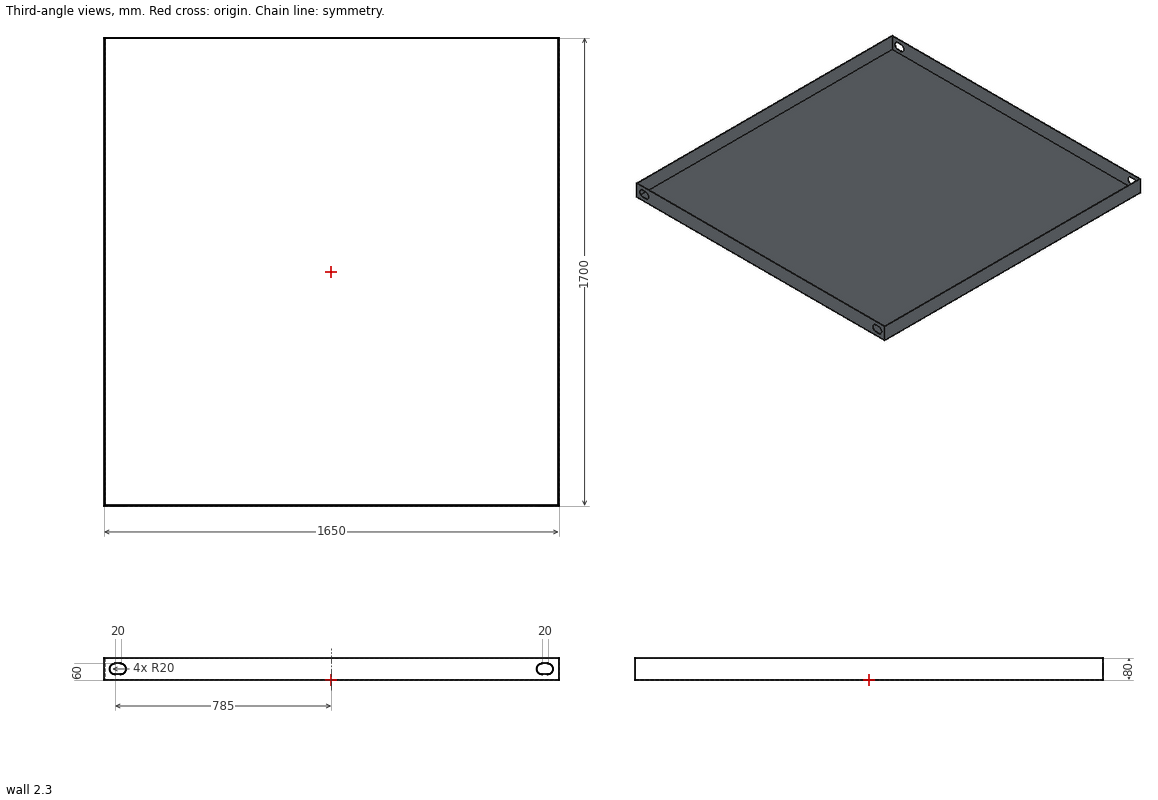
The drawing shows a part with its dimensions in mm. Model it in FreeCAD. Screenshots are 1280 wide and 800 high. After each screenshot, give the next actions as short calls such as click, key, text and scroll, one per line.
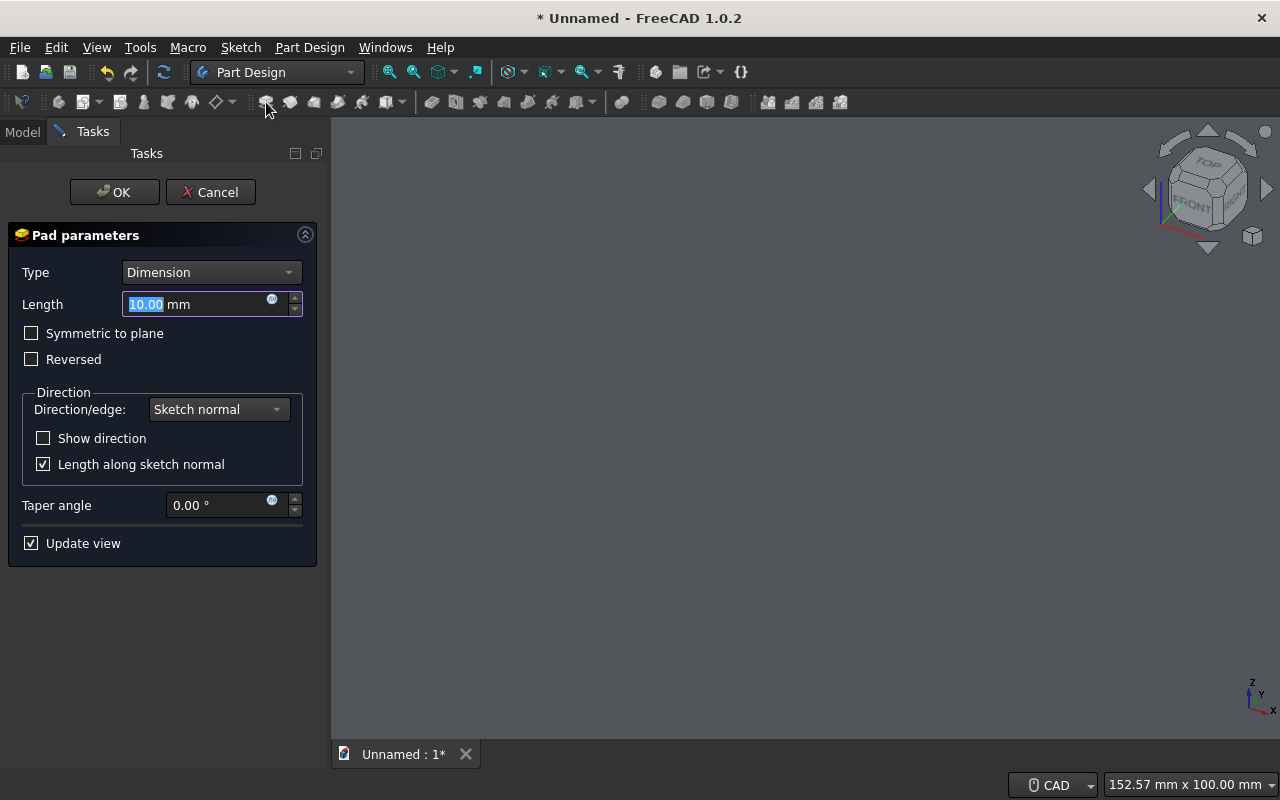
text(80)
key(Tab)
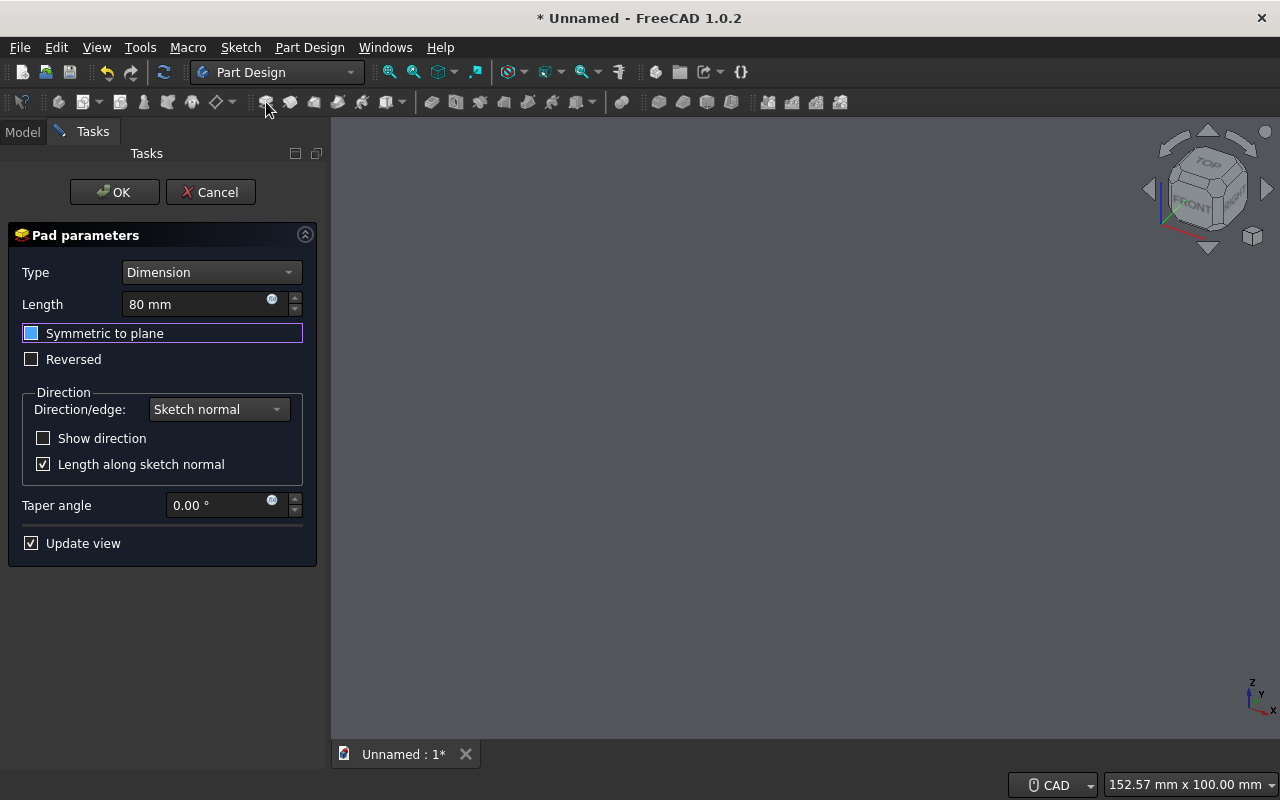
click(115, 192)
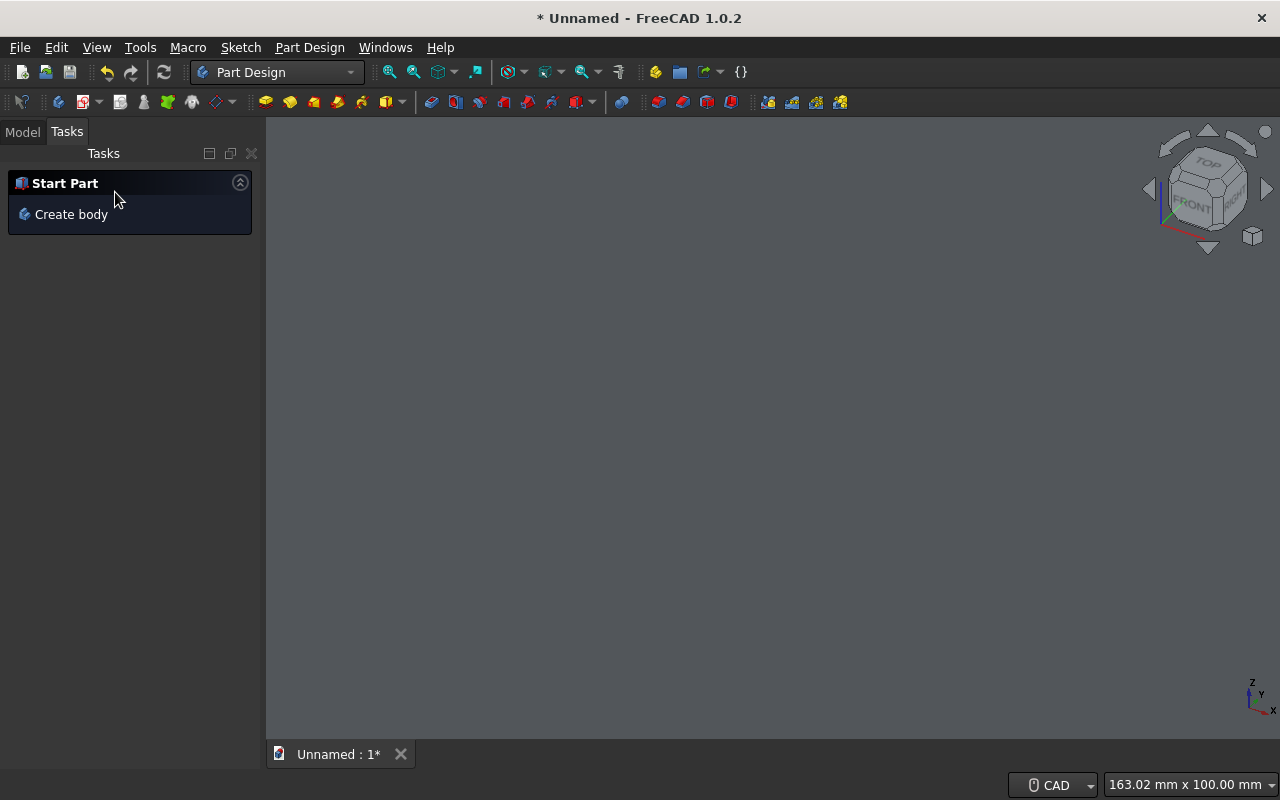
key(v)
key(f)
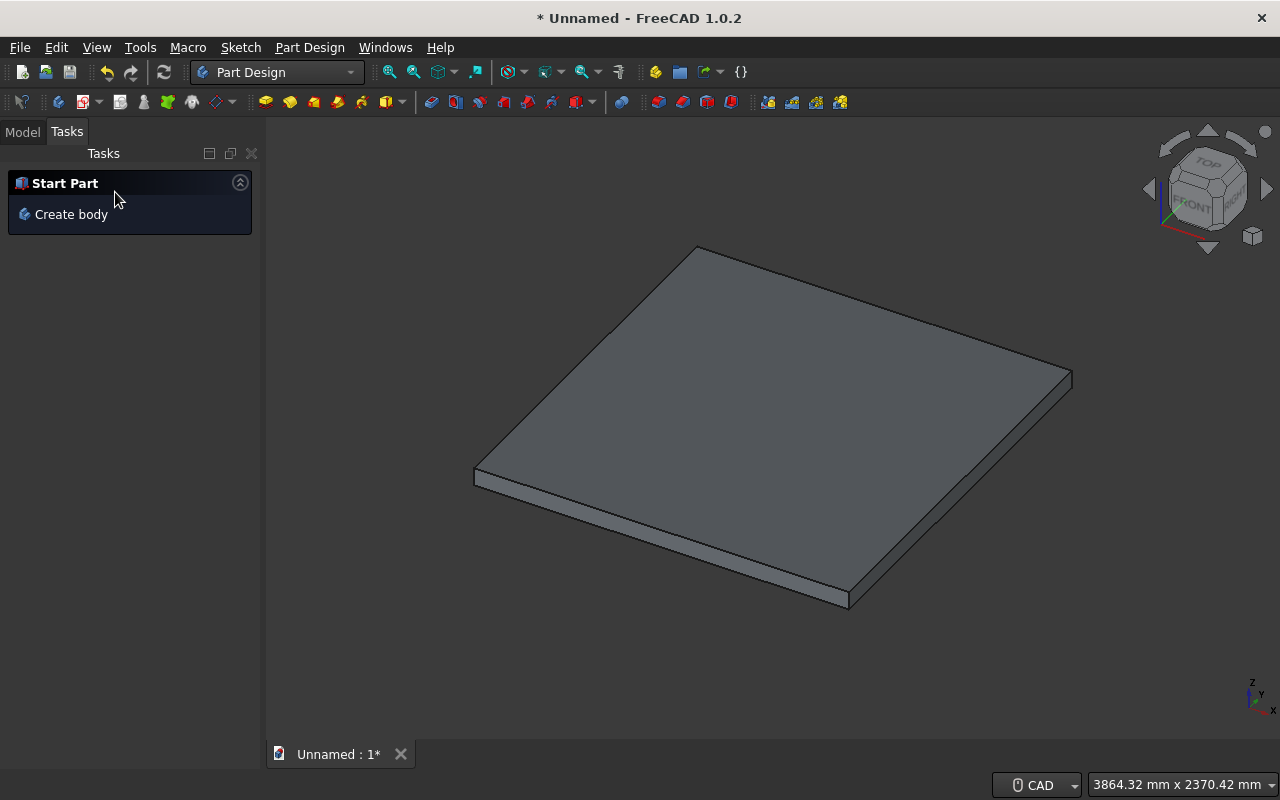
click(773, 418)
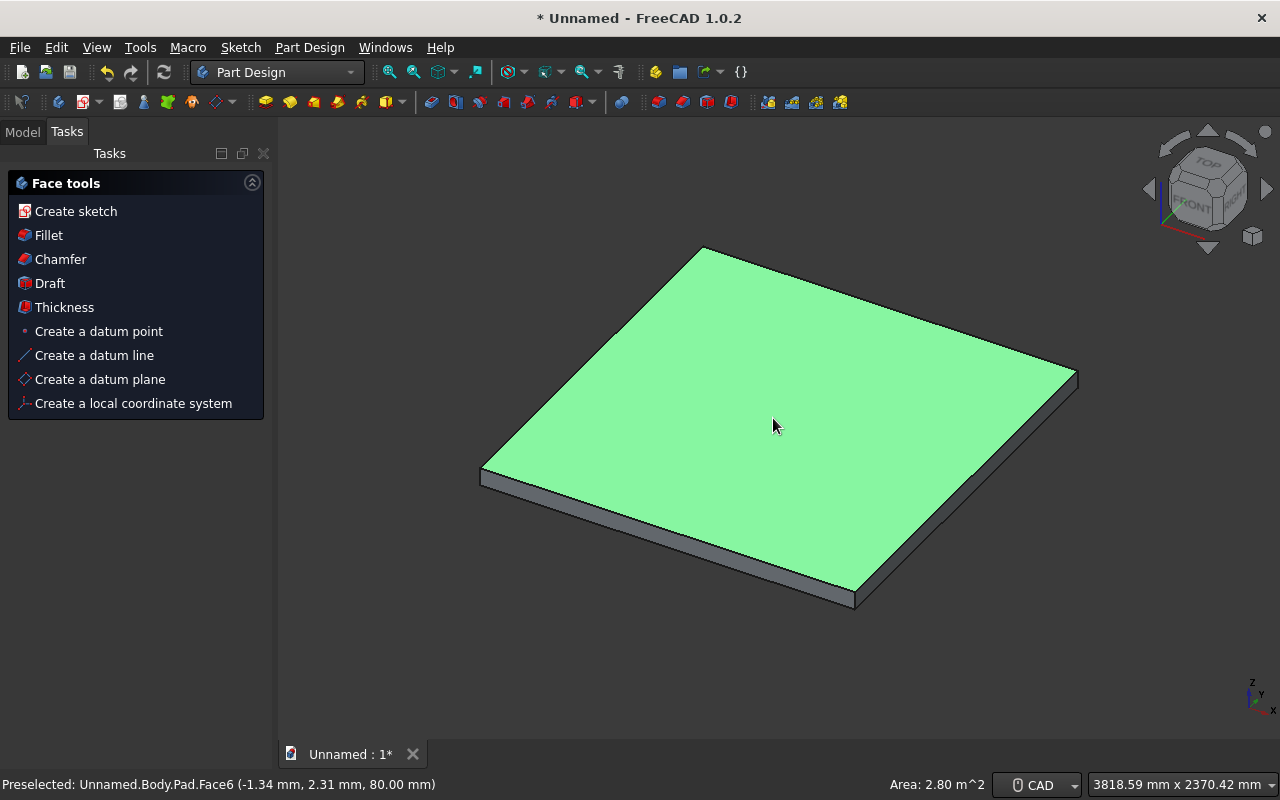
click(732, 102)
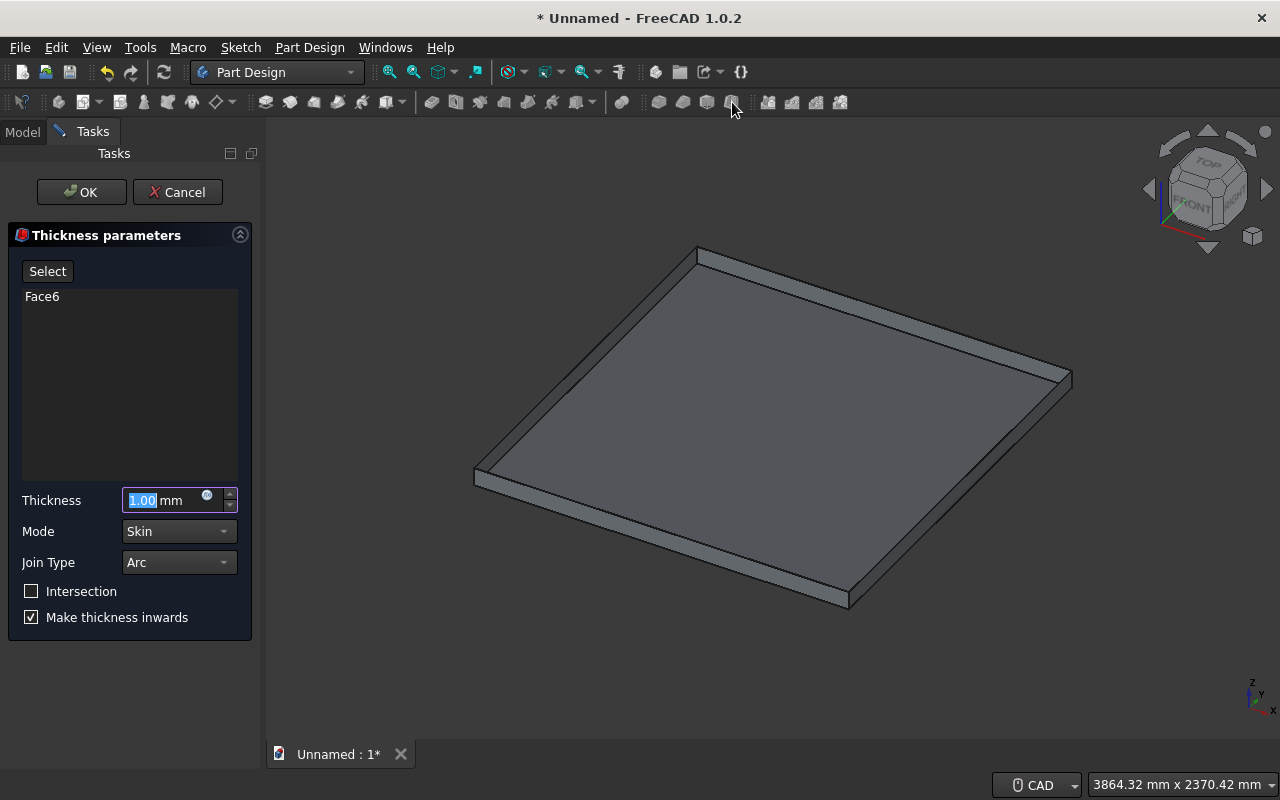
text(2.3)
key(Tab)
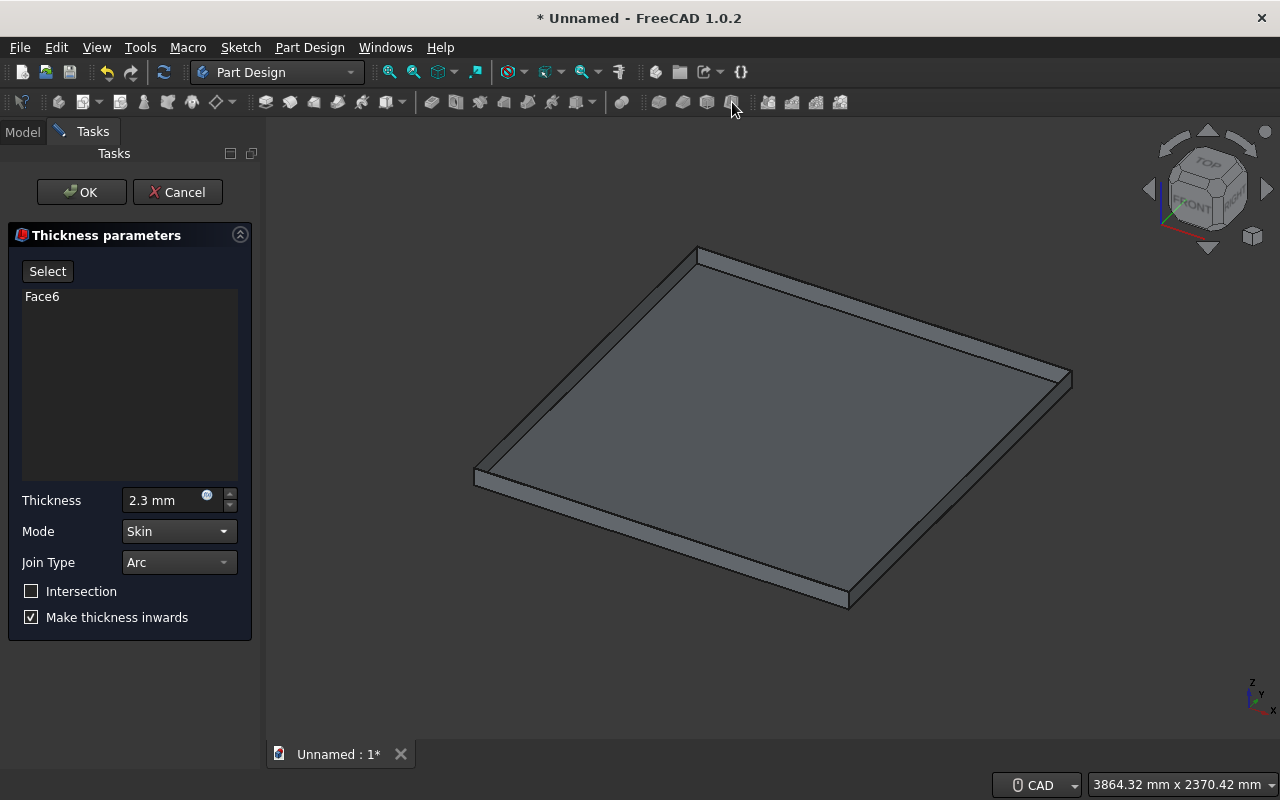
click(180, 562)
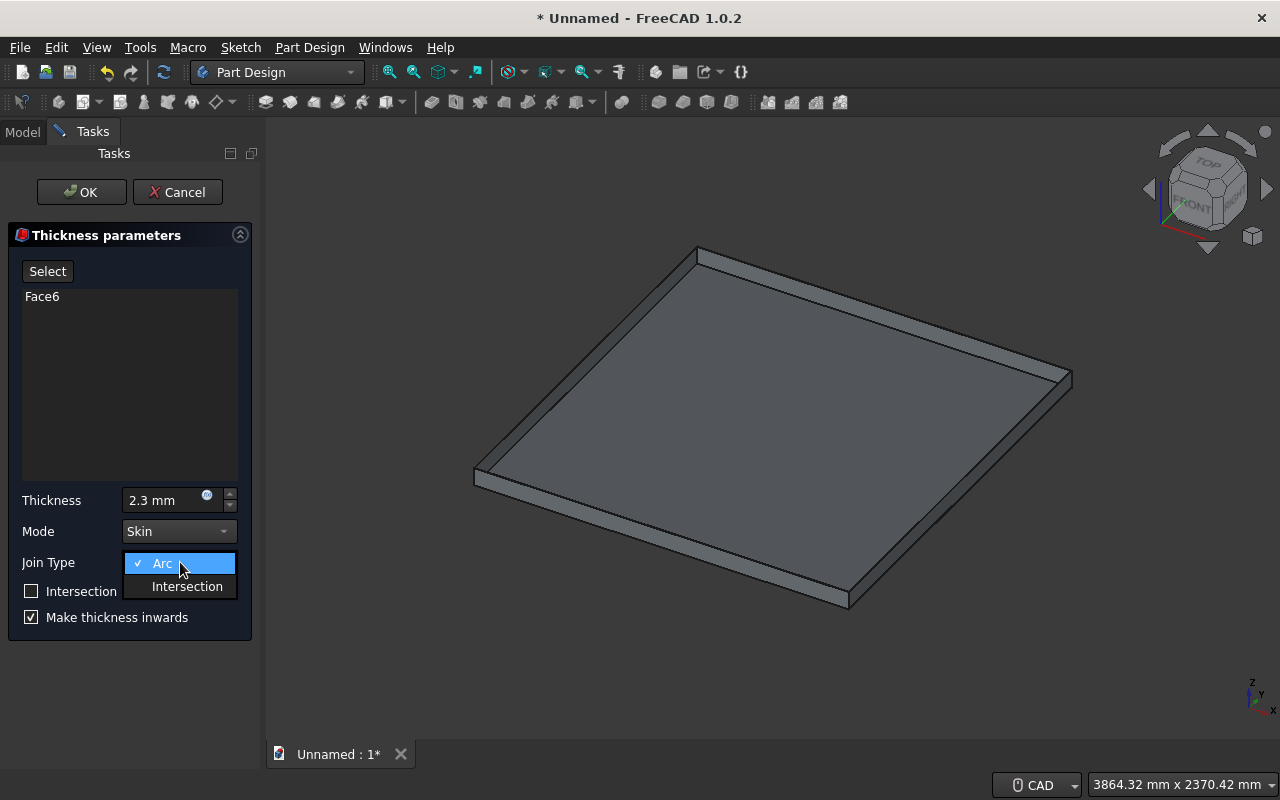
click(179, 586)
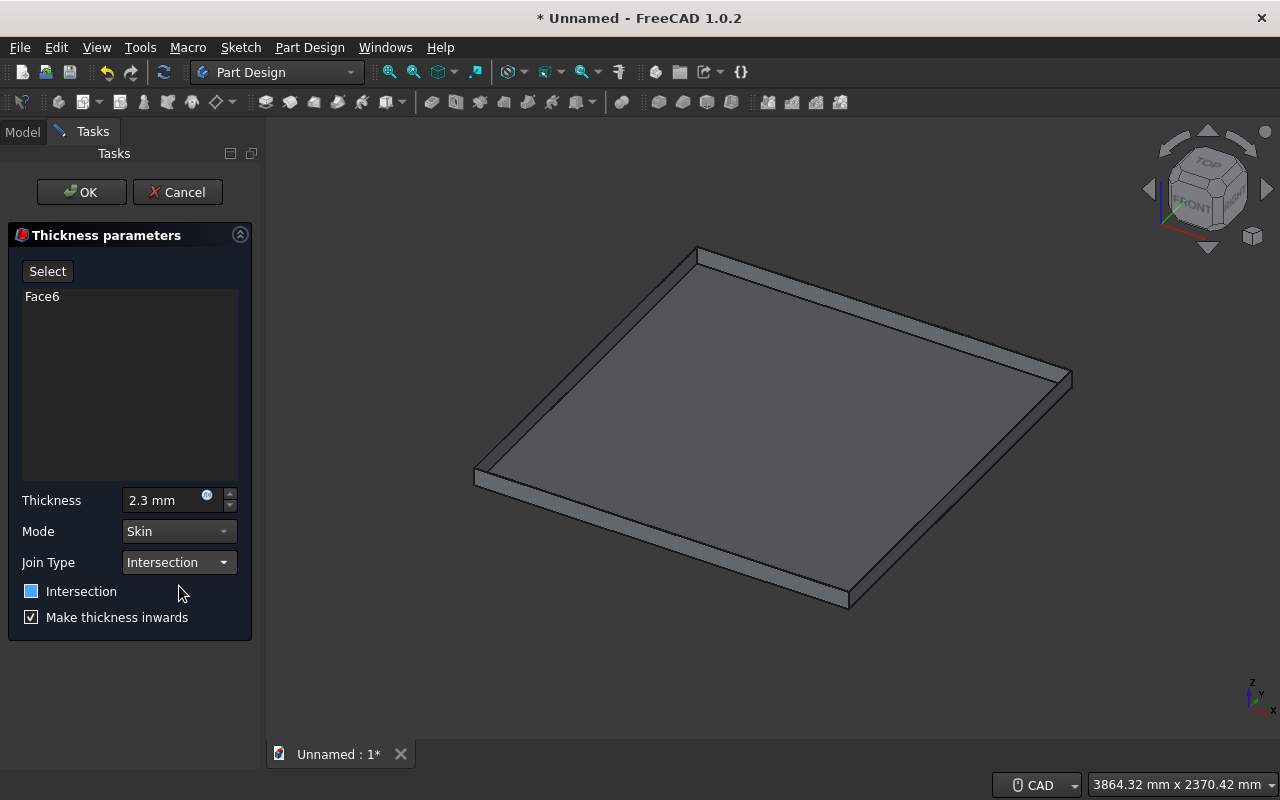
click(82, 192)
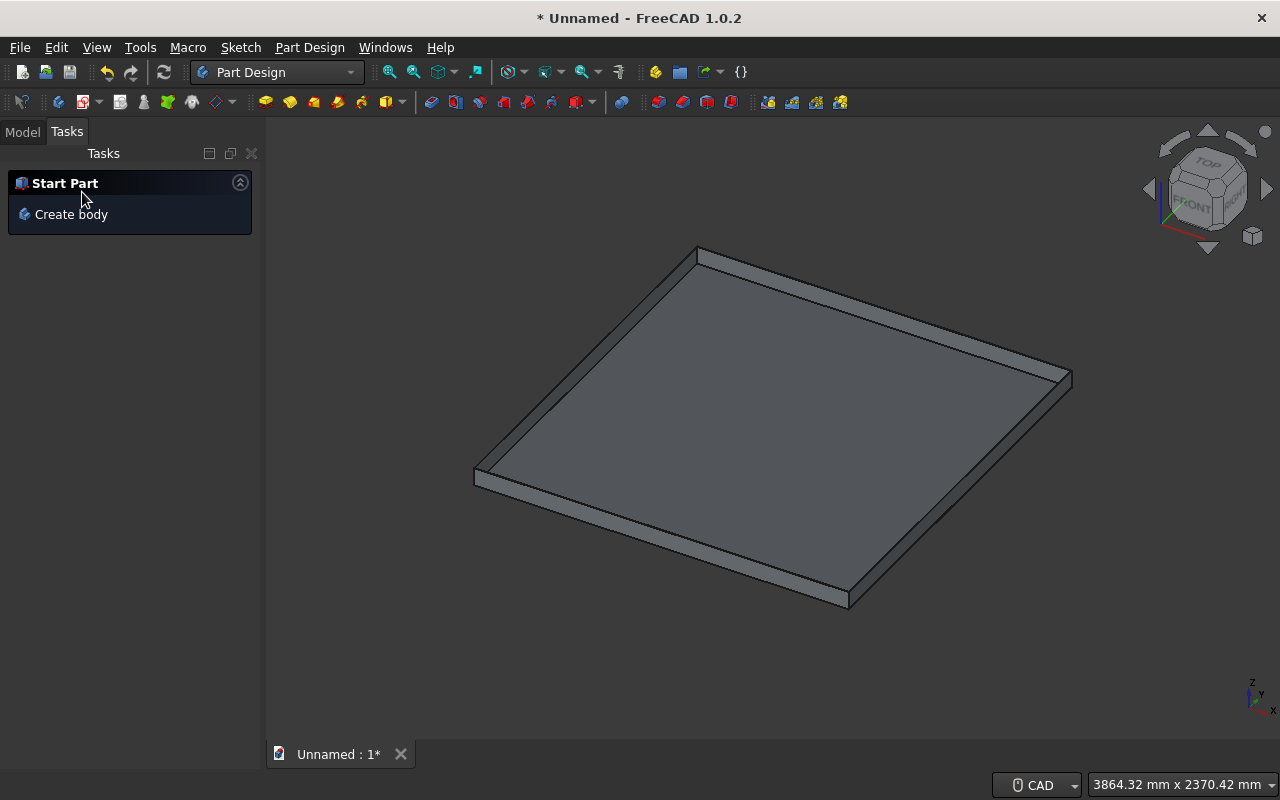
key(0)